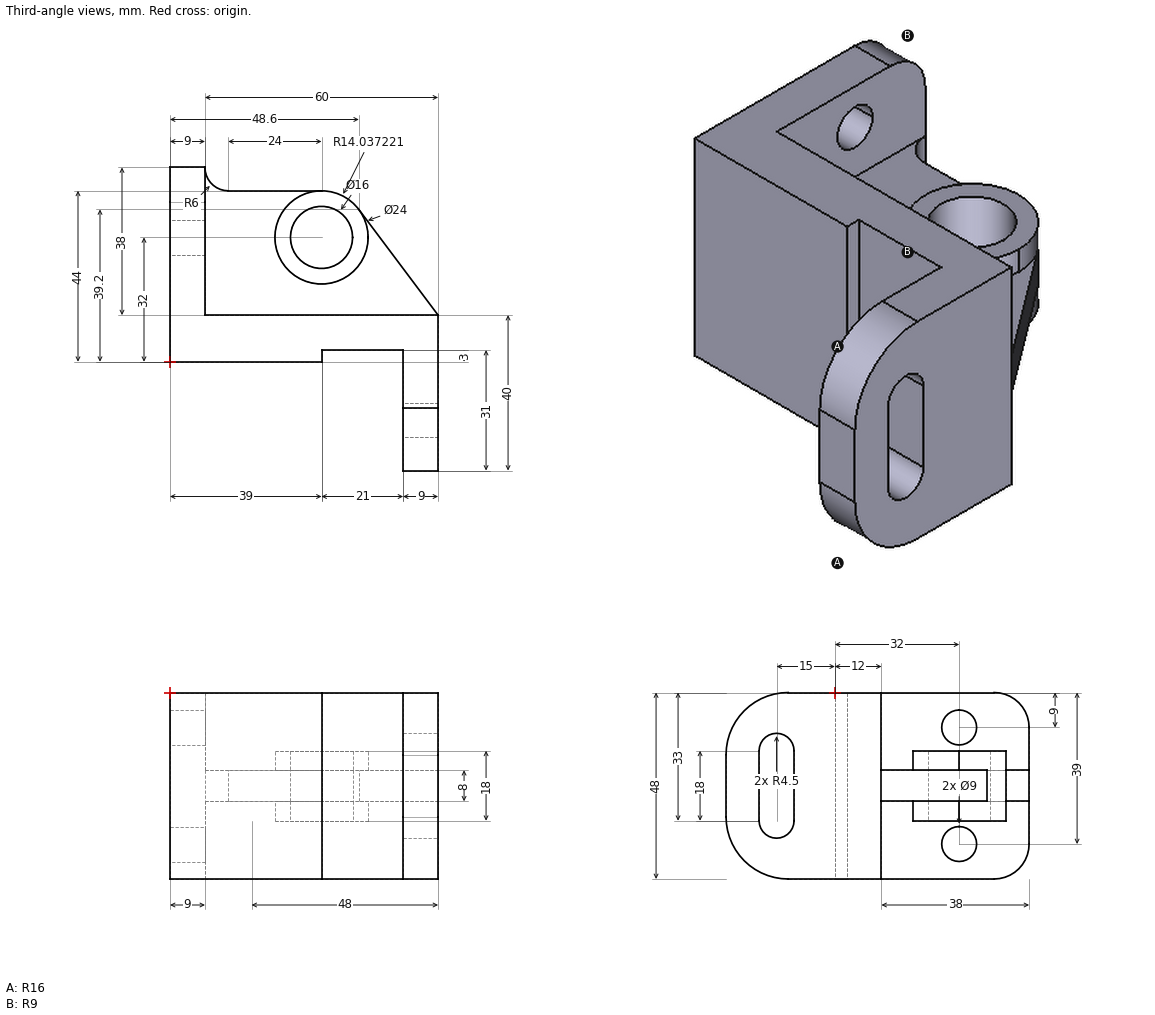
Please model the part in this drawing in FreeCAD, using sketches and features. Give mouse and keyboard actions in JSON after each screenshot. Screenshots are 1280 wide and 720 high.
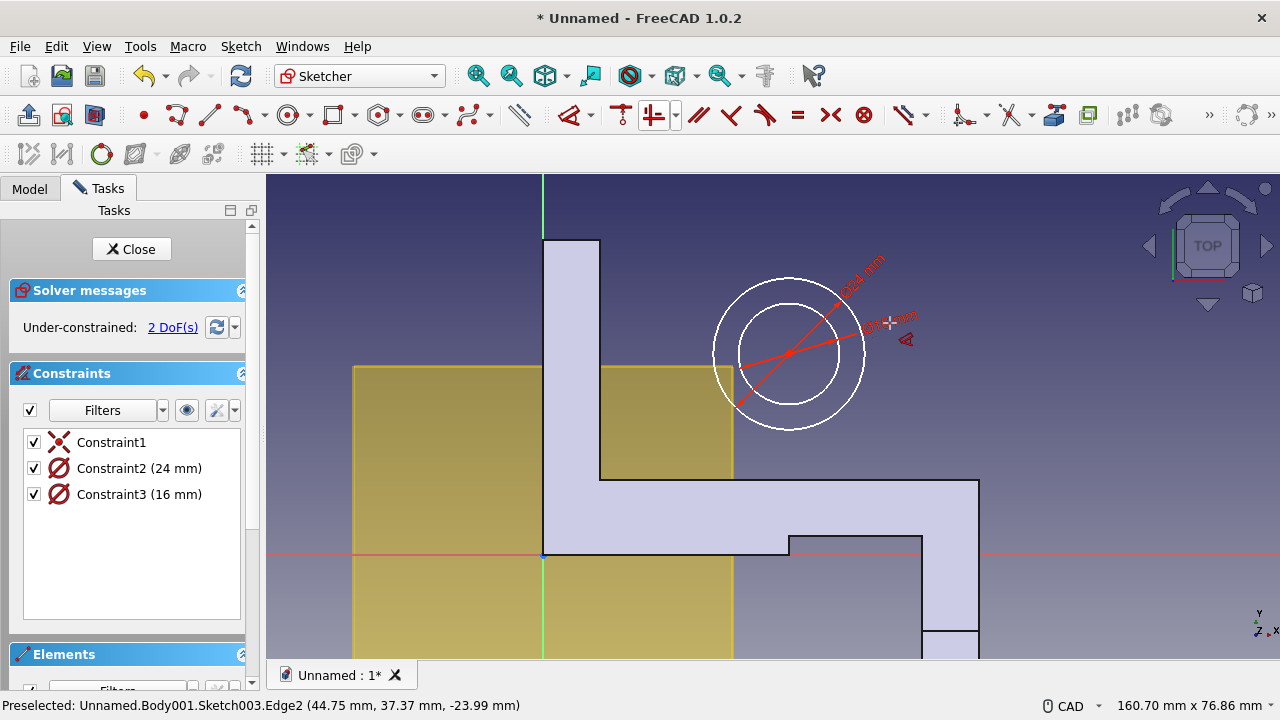
{"action": "left_click", "coordinate": [789, 354]}
{"action": "left_click", "coordinate": [666, 589]}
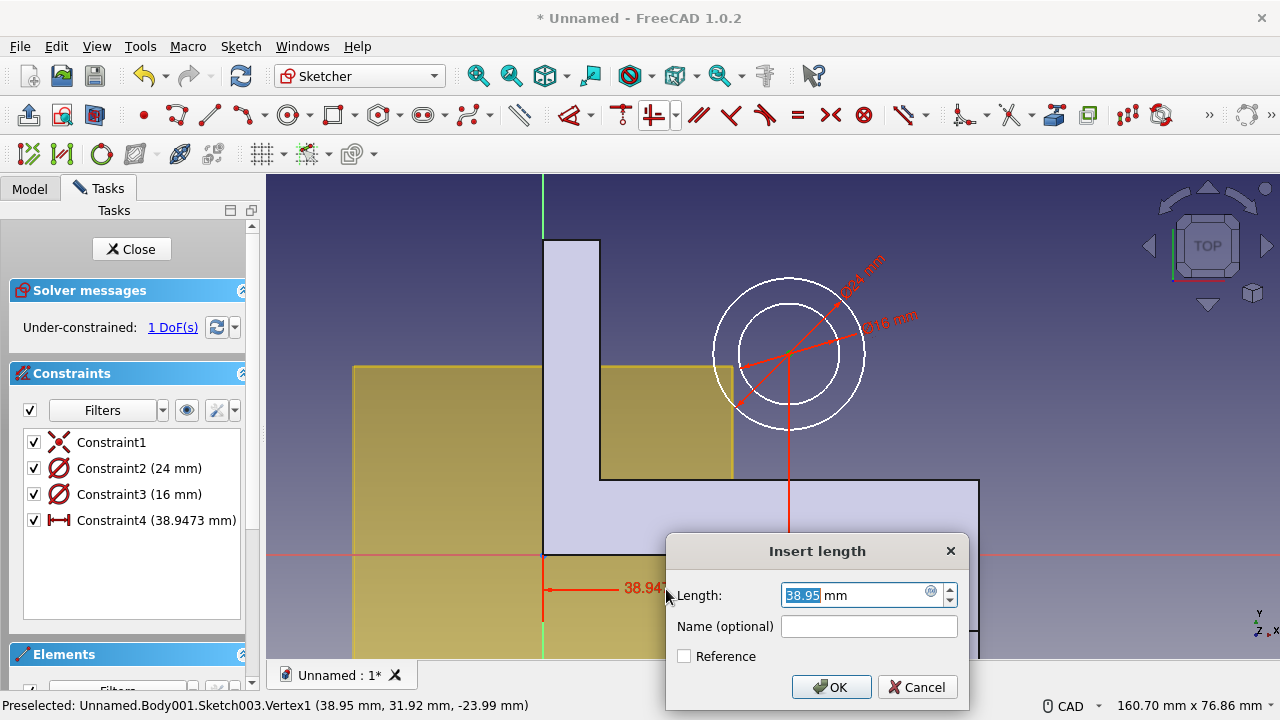
{"action": "type", "text": "39"}
{"action": "key", "text": "Return"}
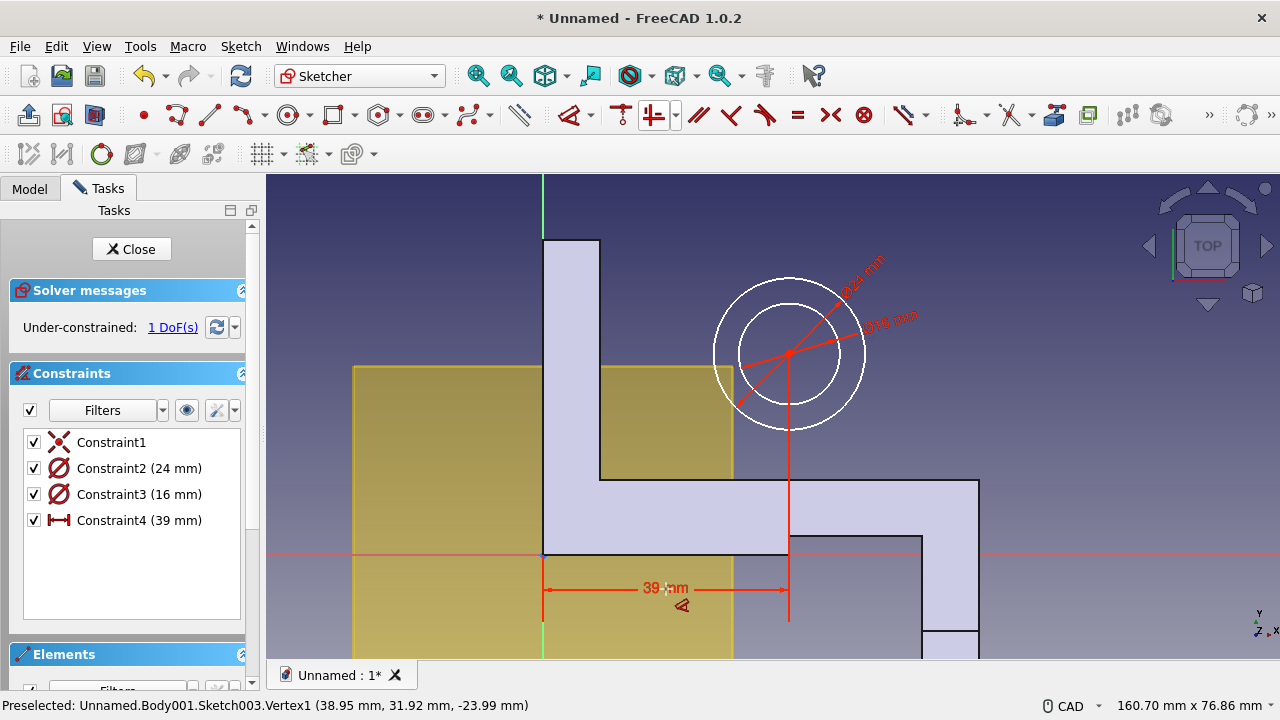
{"action": "left_click", "coordinate": [789, 354]}
{"action": "left_click", "coordinate": [509, 455]}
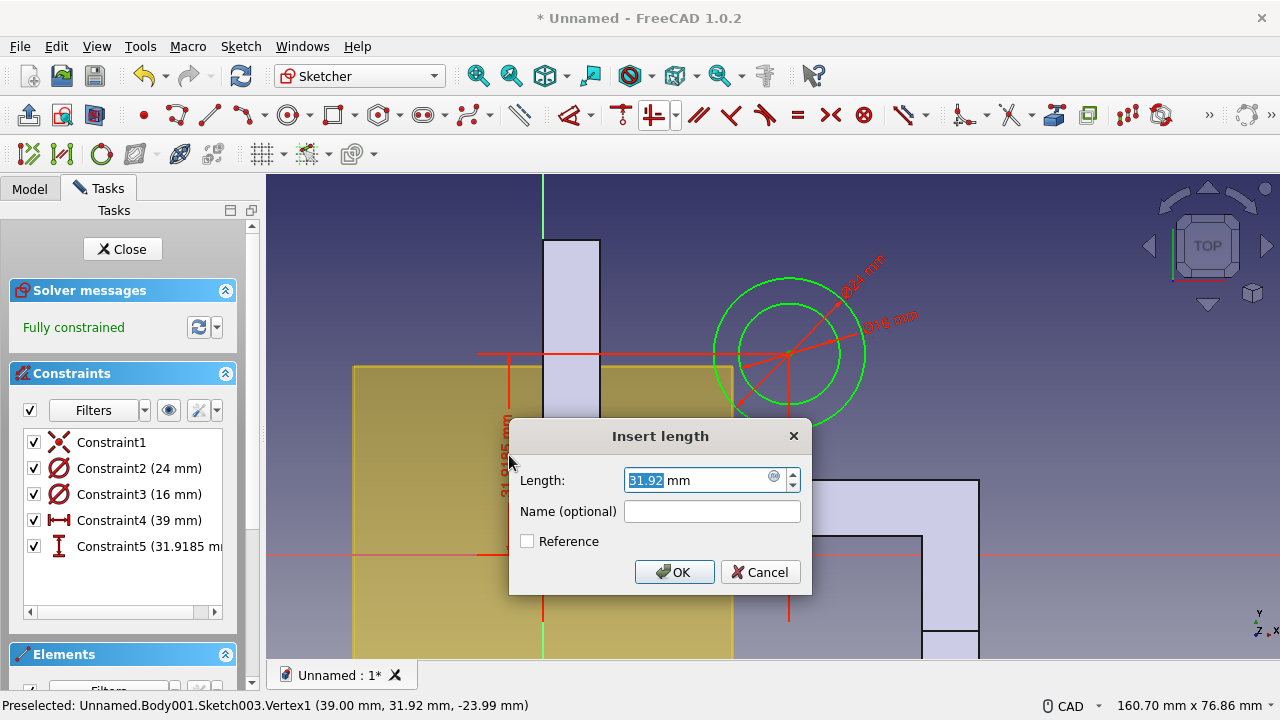
{"action": "type", "text": "32"}
{"action": "key", "text": "Return"}
{"action": "key", "text": "Escape"}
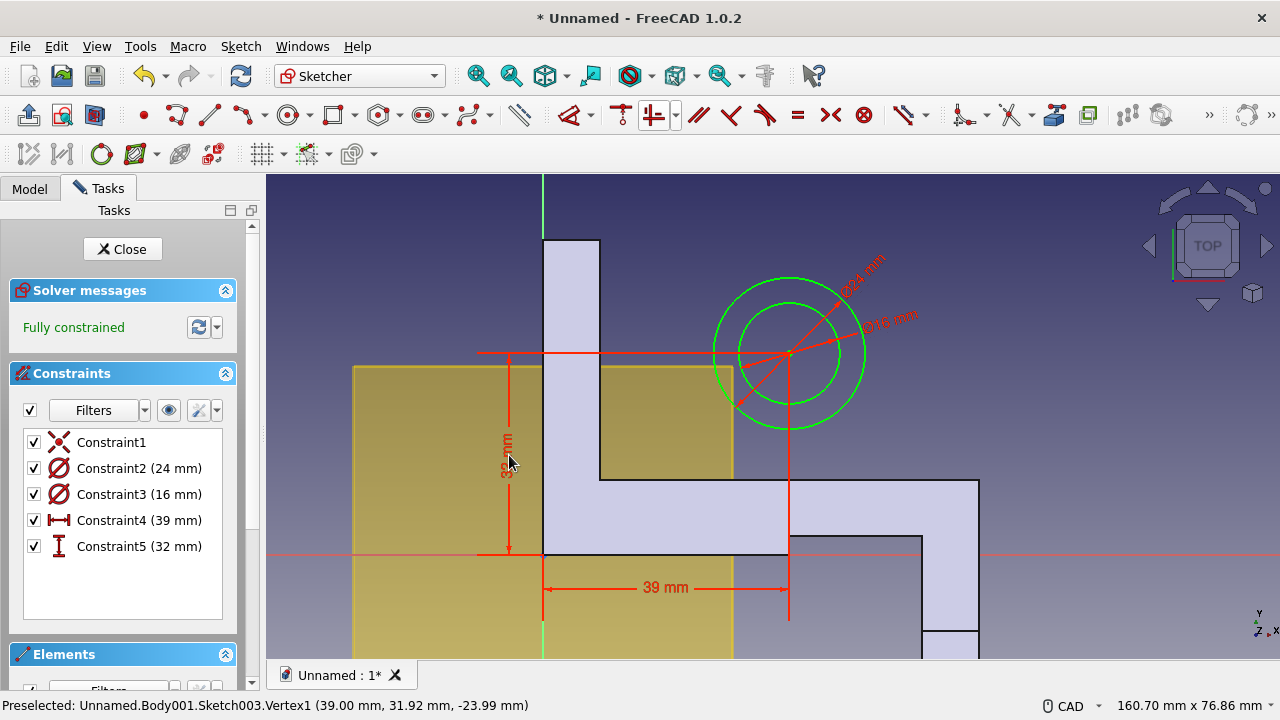
{"action": "left_click", "coordinate": [123, 249]}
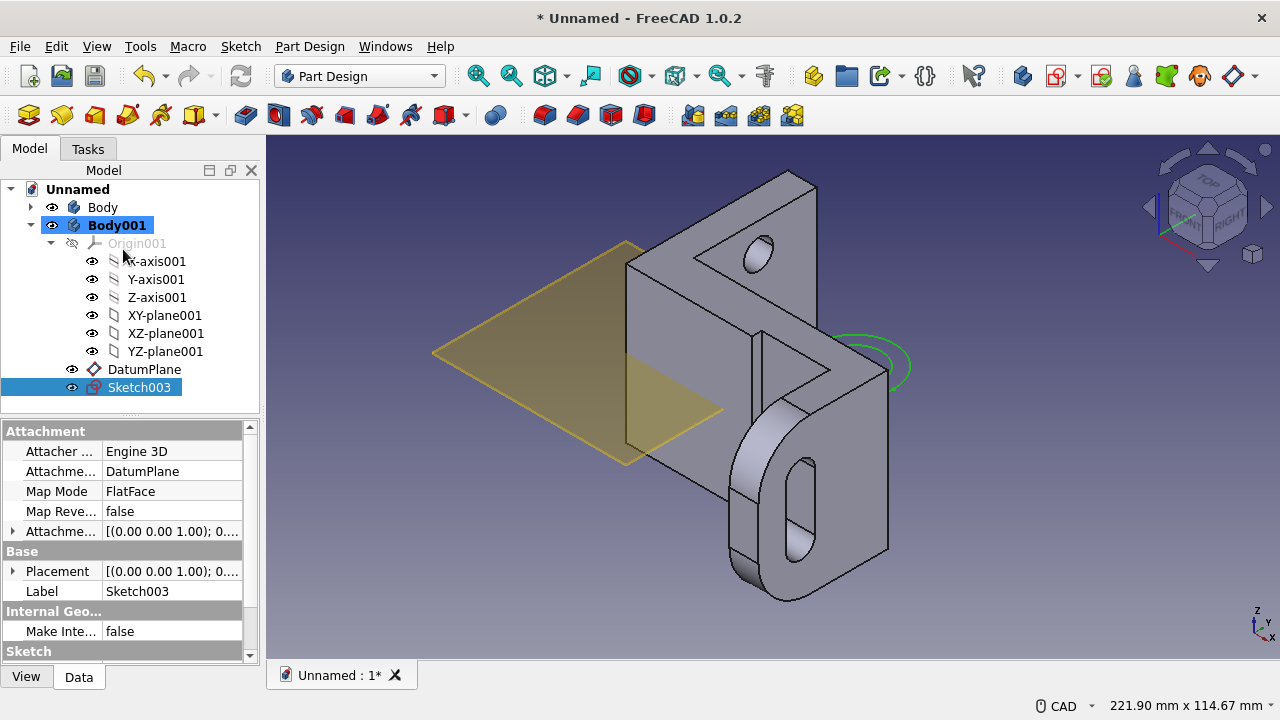
{"action": "left_click", "coordinate": [29, 116]}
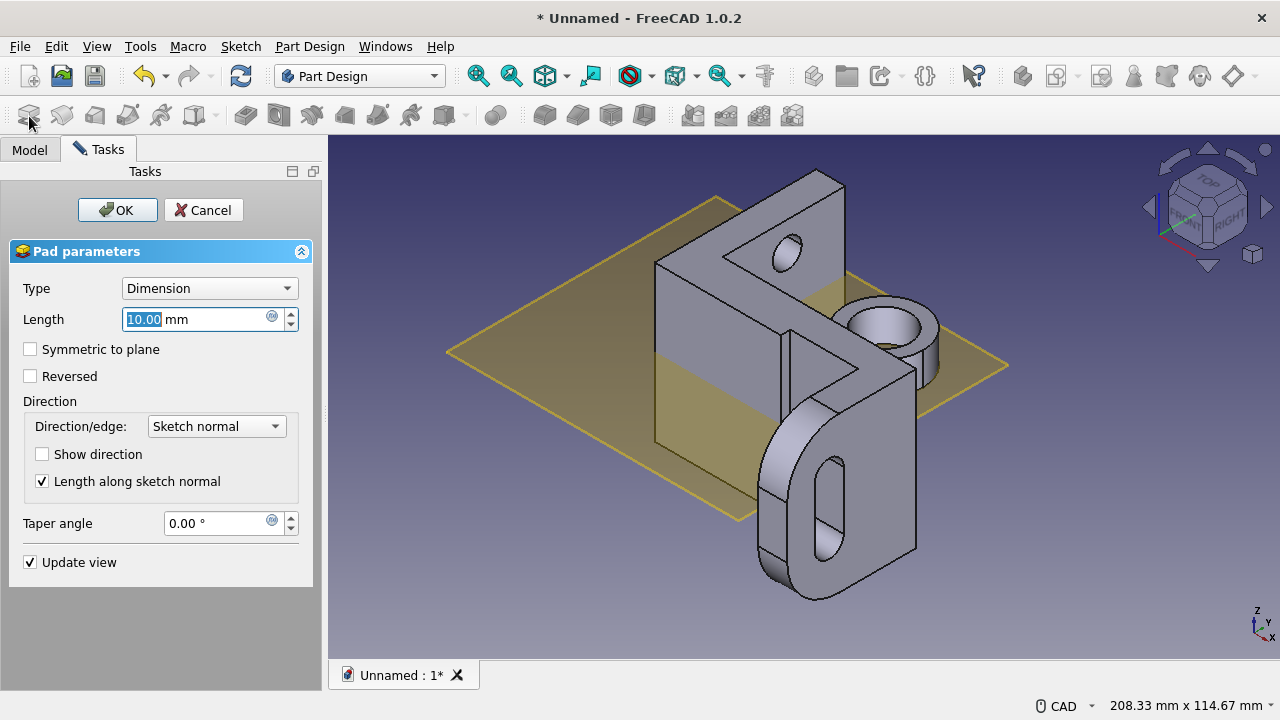
{"action": "type", "text": "18"}
{"action": "key", "text": "Tab"}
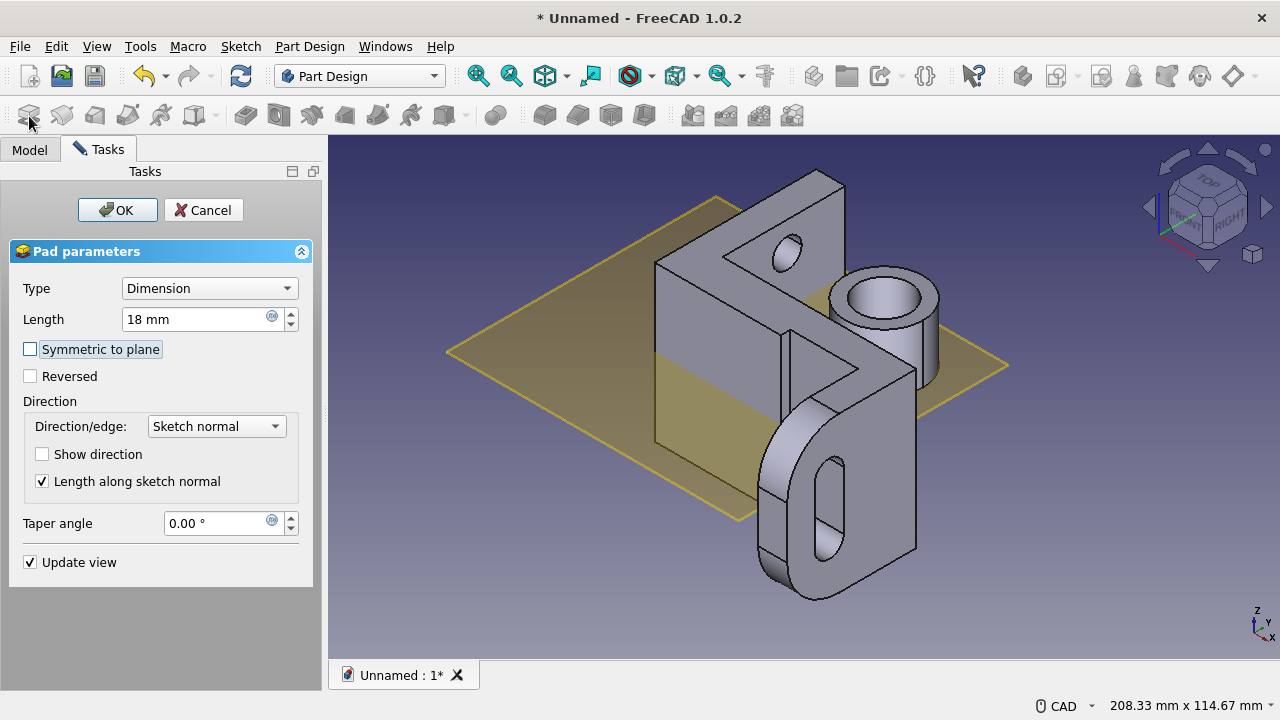
{"action": "left_click", "coordinate": [31, 349]}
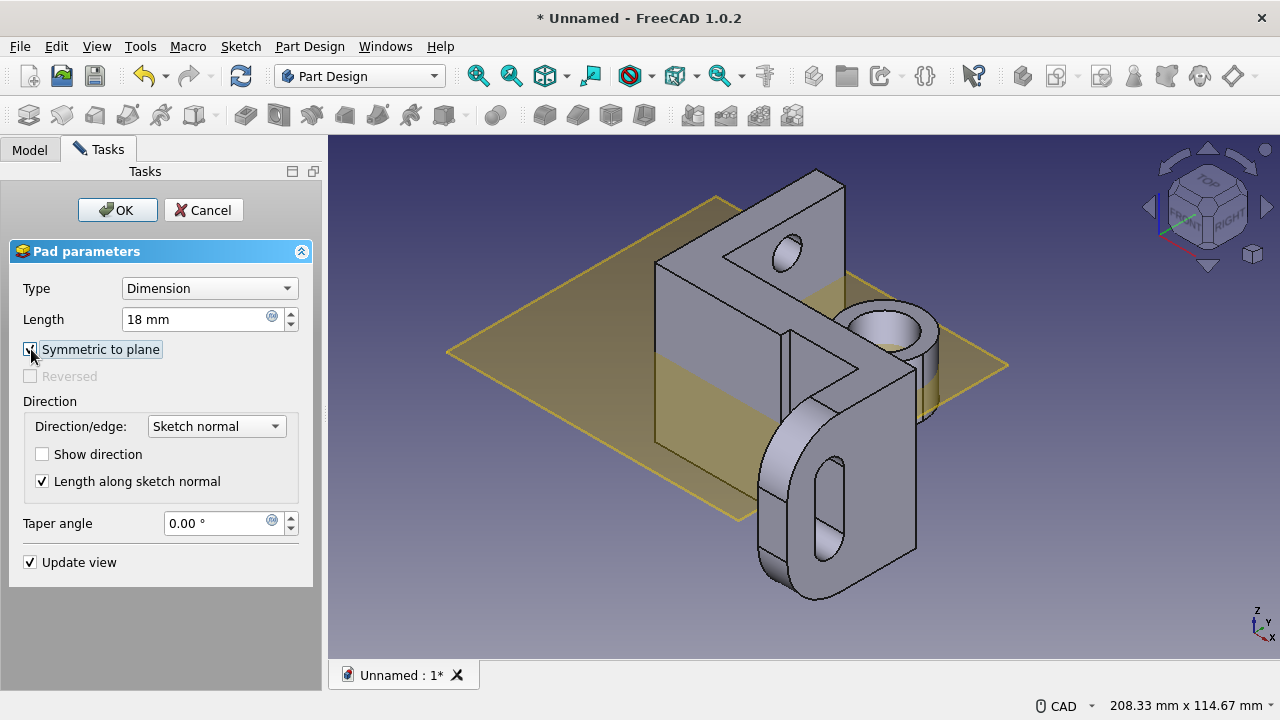
{"action": "left_click", "coordinate": [118, 210]}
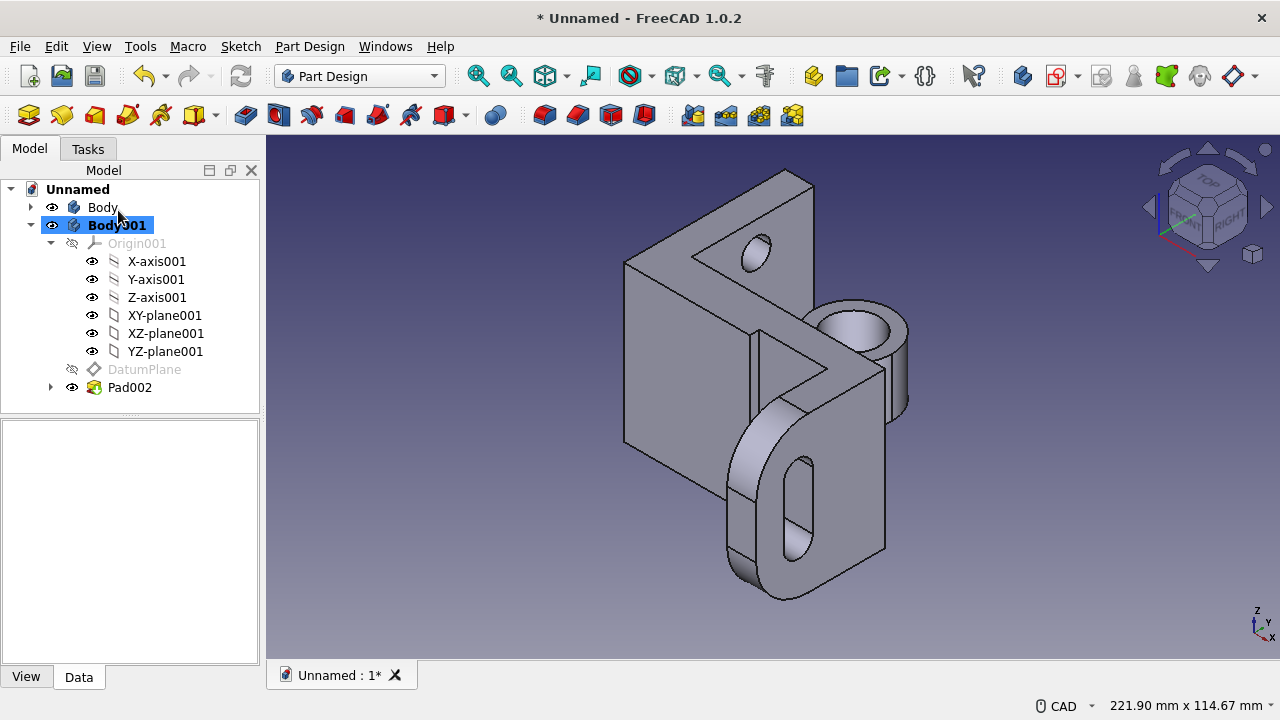
{"action": "left_click", "coordinate": [479, 76]}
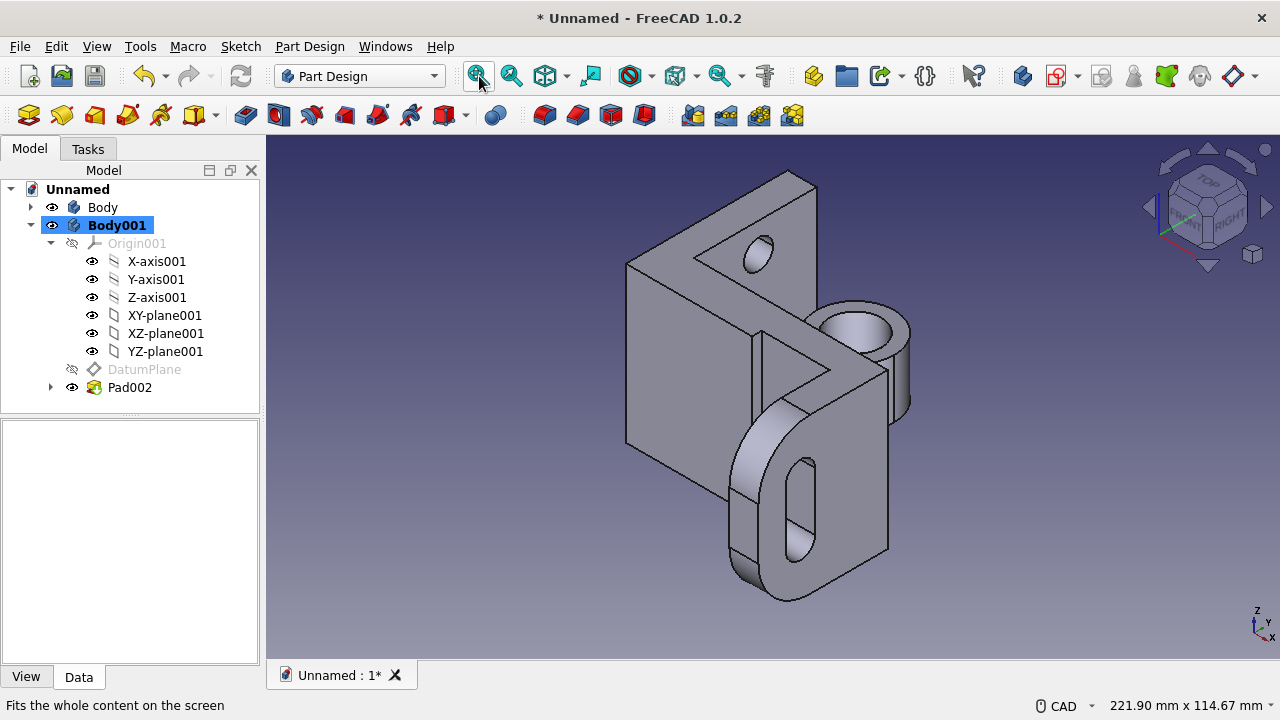
{"action": "double_click", "coordinate": [97, 207]}